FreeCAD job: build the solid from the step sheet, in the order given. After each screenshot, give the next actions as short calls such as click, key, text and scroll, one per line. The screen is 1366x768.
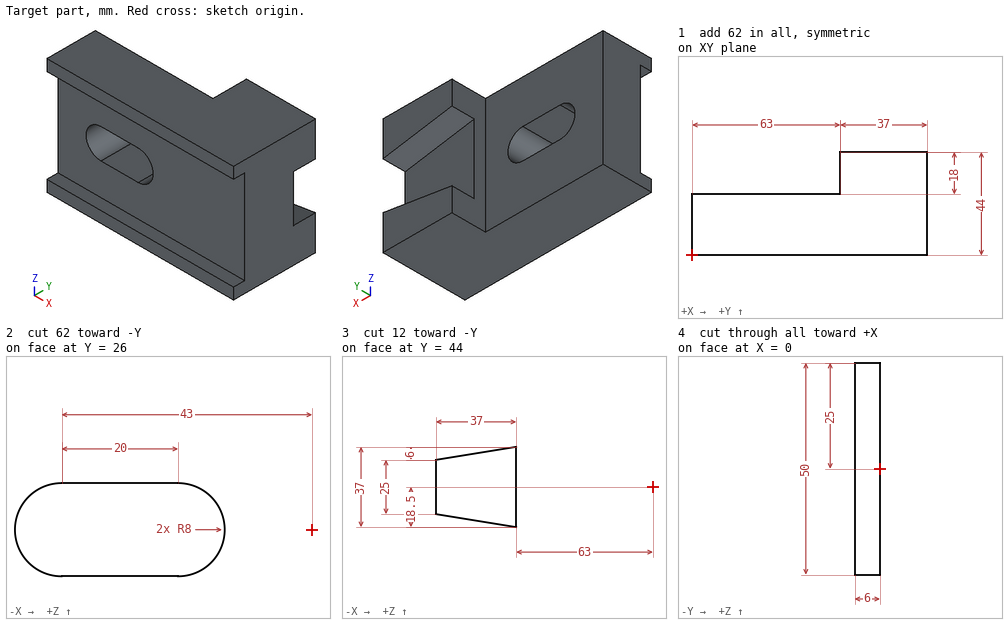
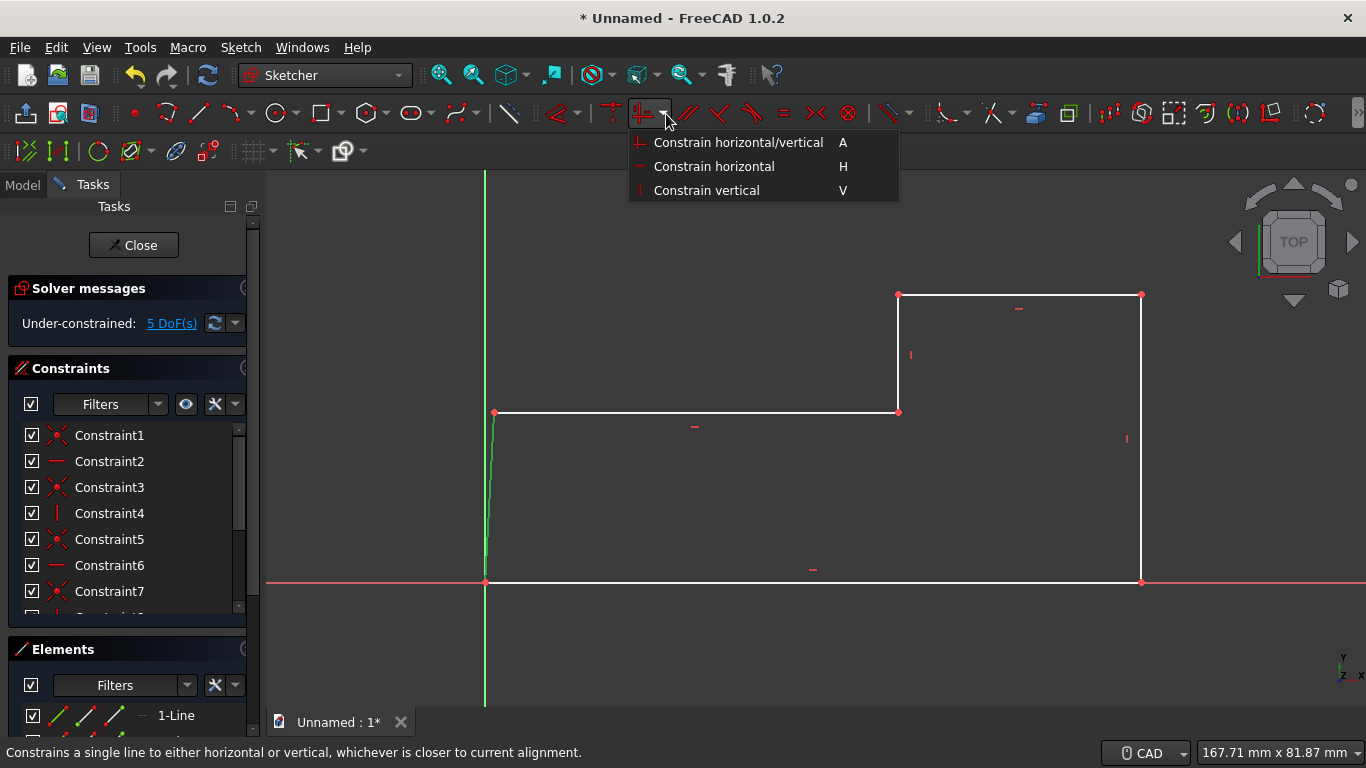
click(764, 190)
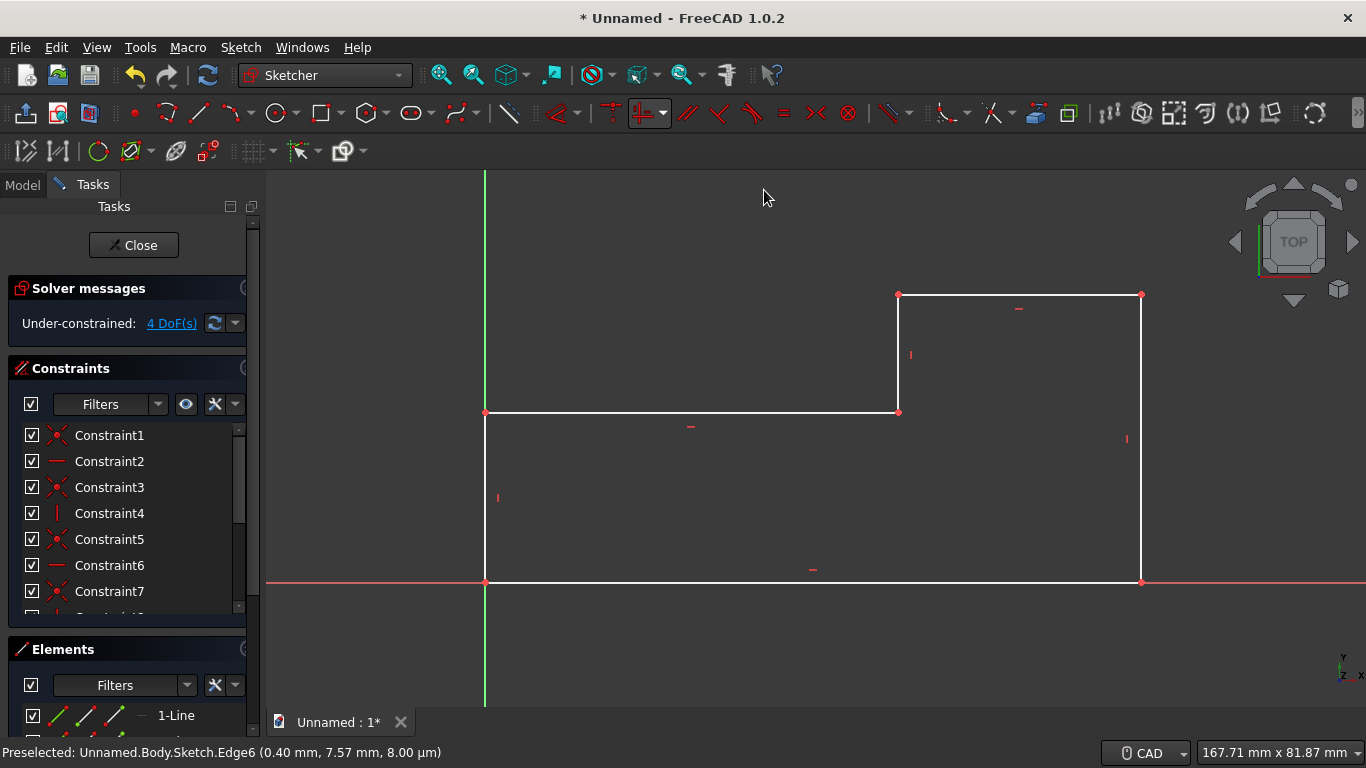
click(556, 114)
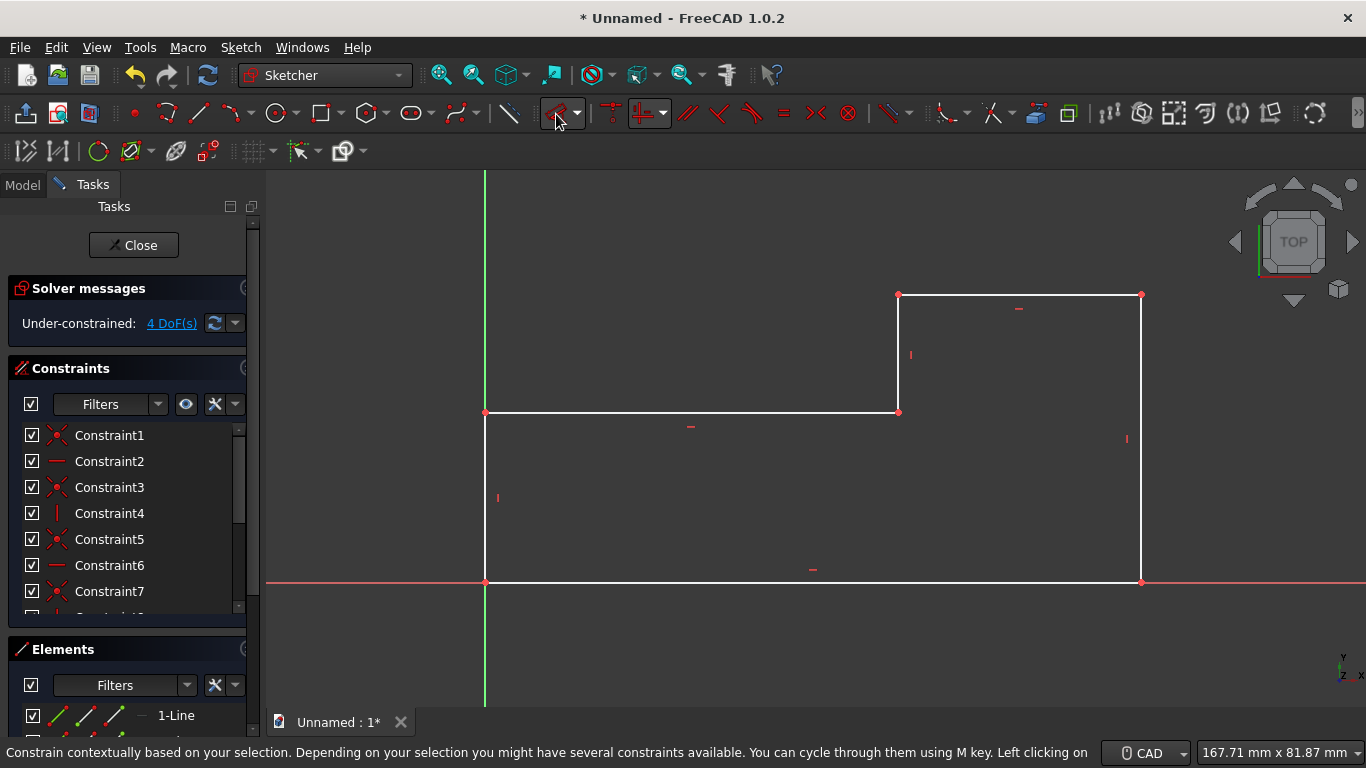
click(1141, 496)
click(1175, 439)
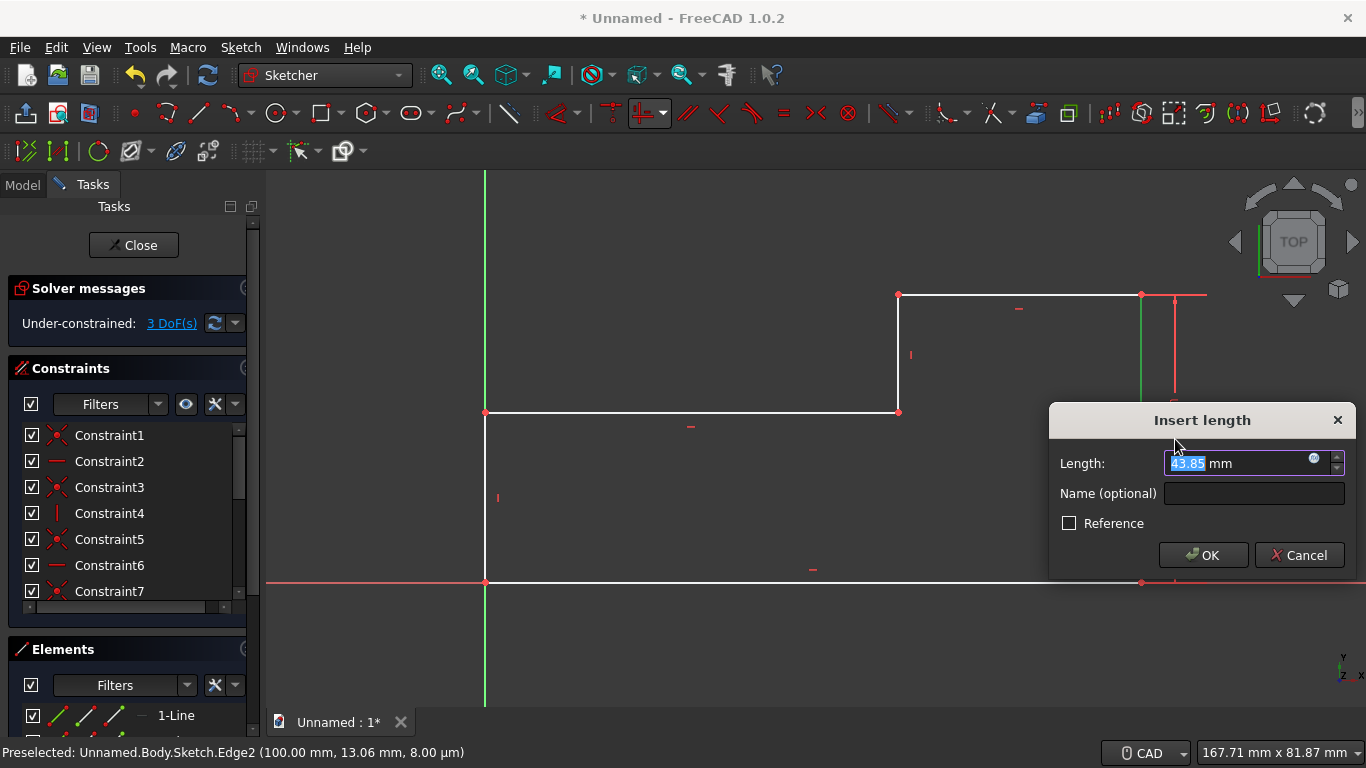
text(44)
key(Return)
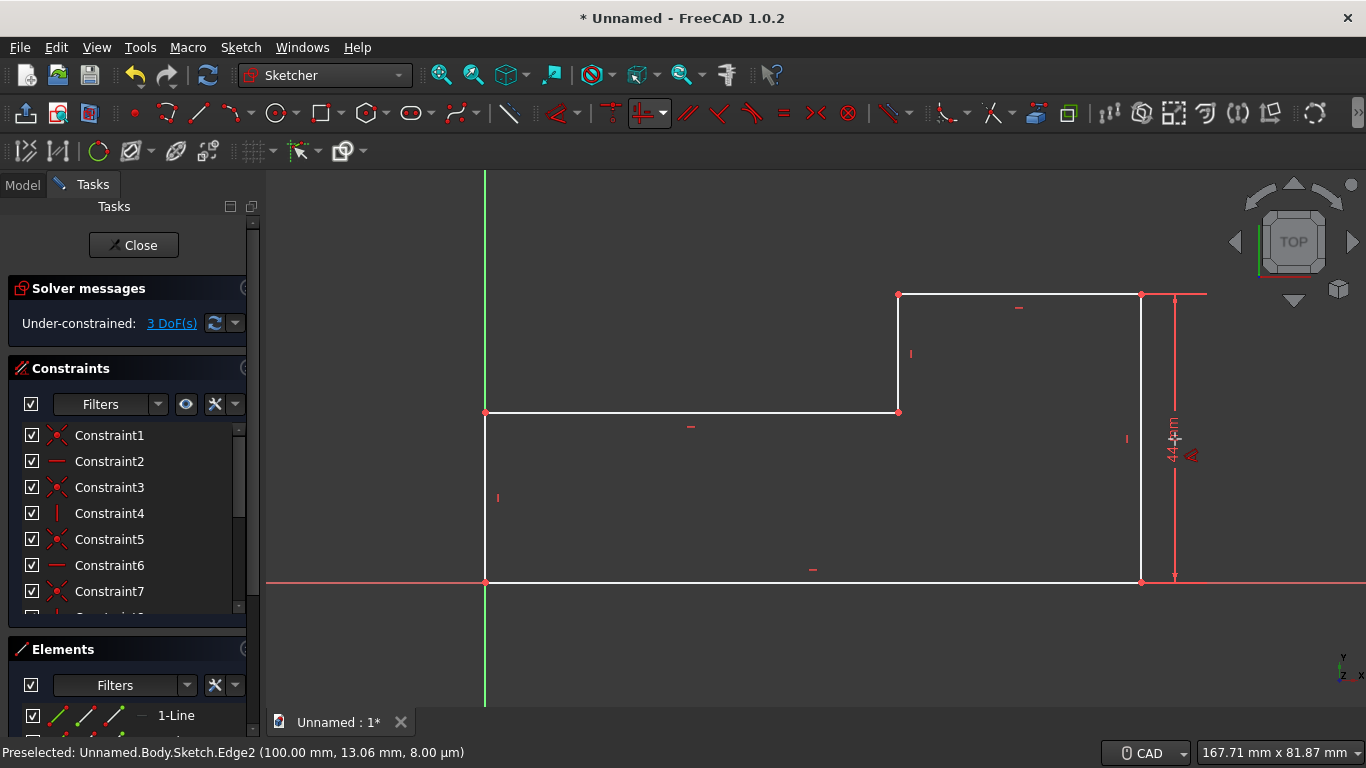
click(1068, 294)
click(1019, 260)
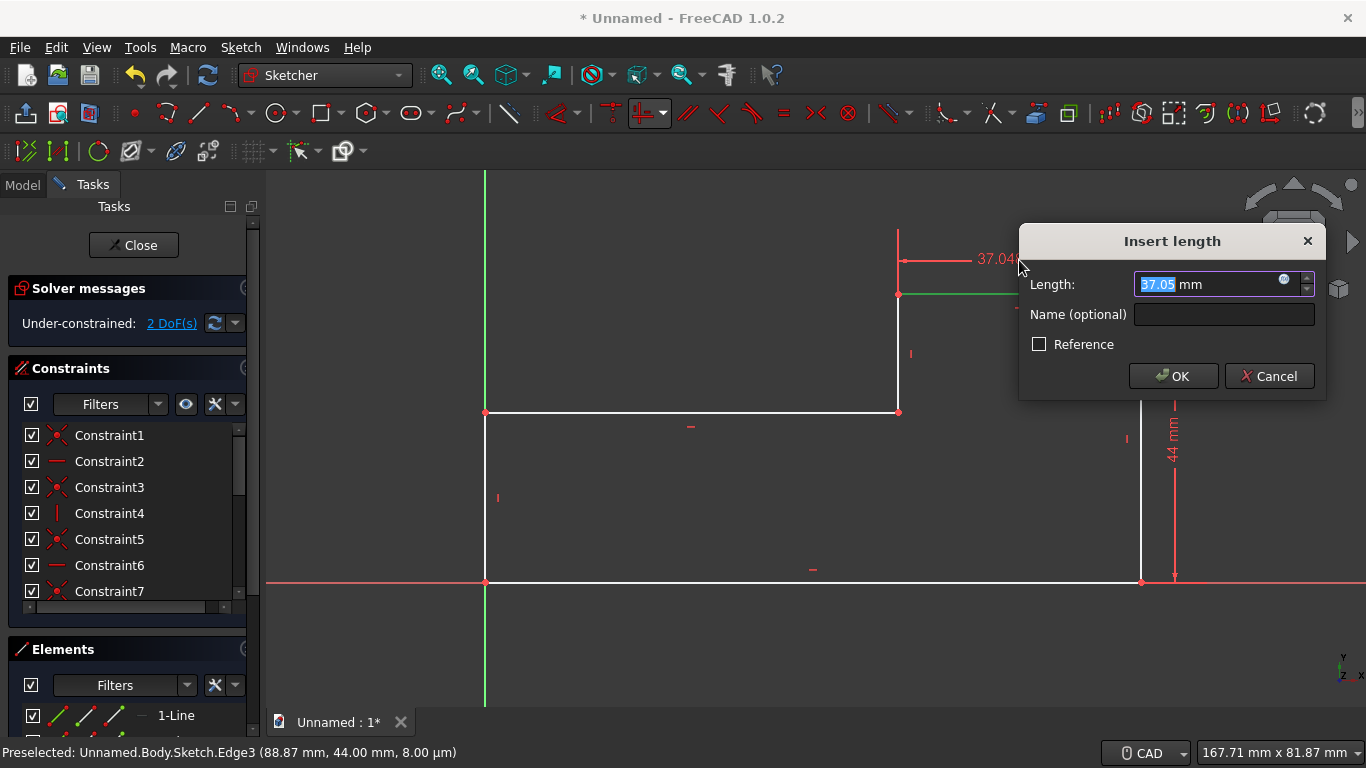
text(37)
key(Return)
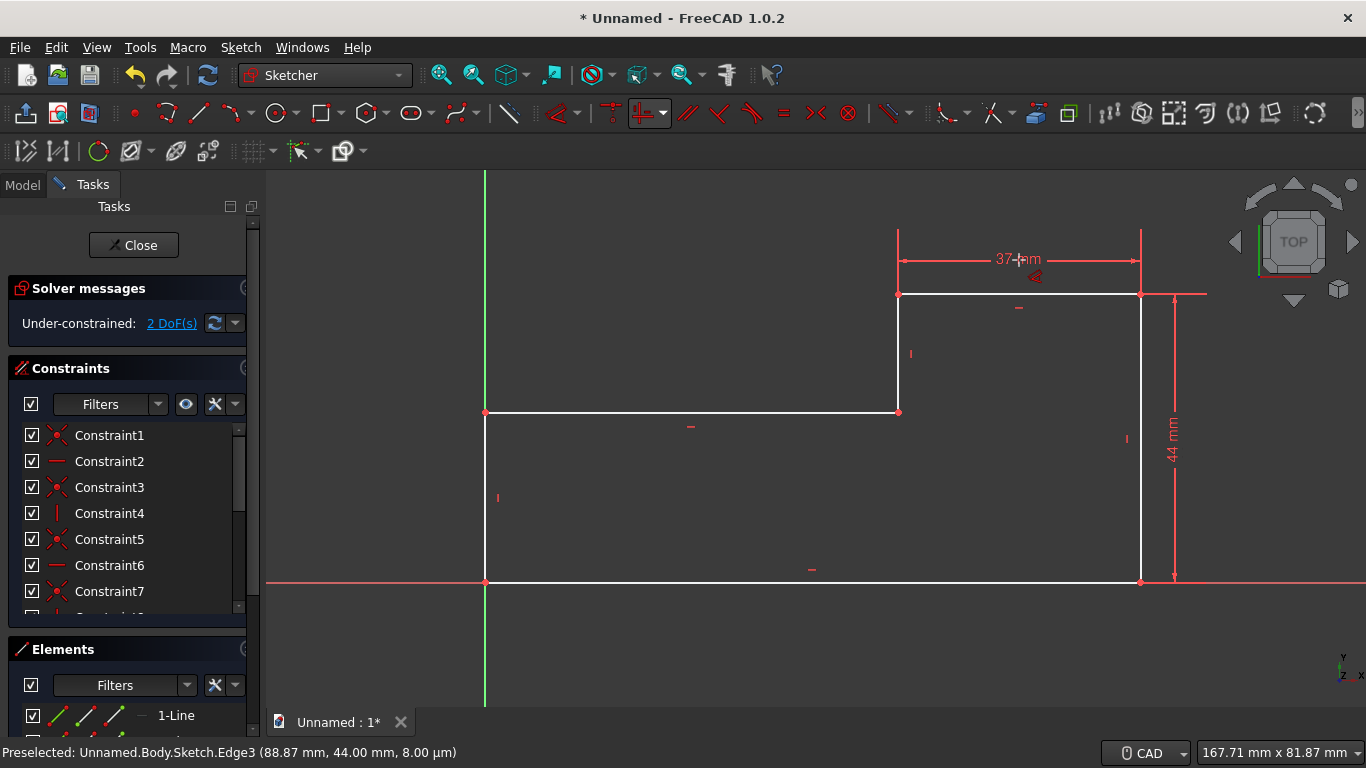
click(898, 330)
click(932, 354)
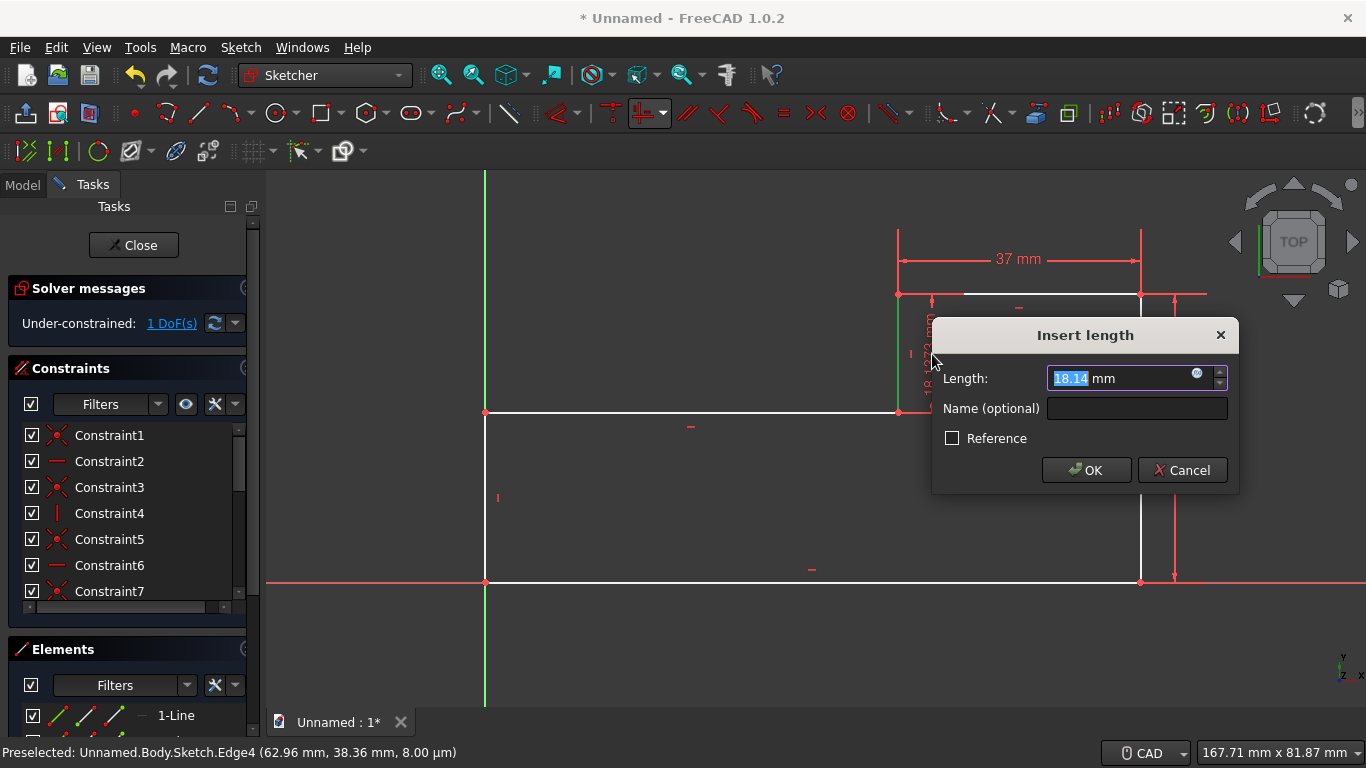
text(18)
key(Return)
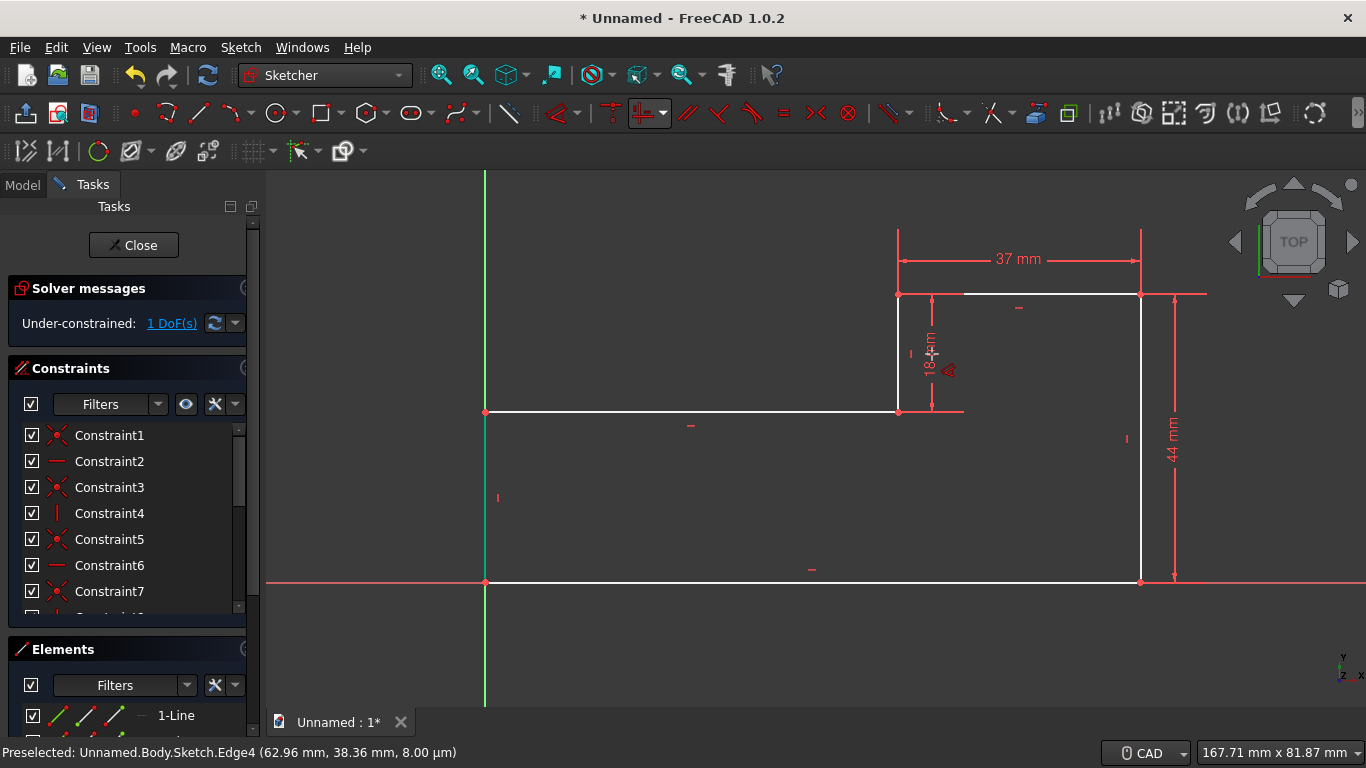
click(774, 412)
click(692, 378)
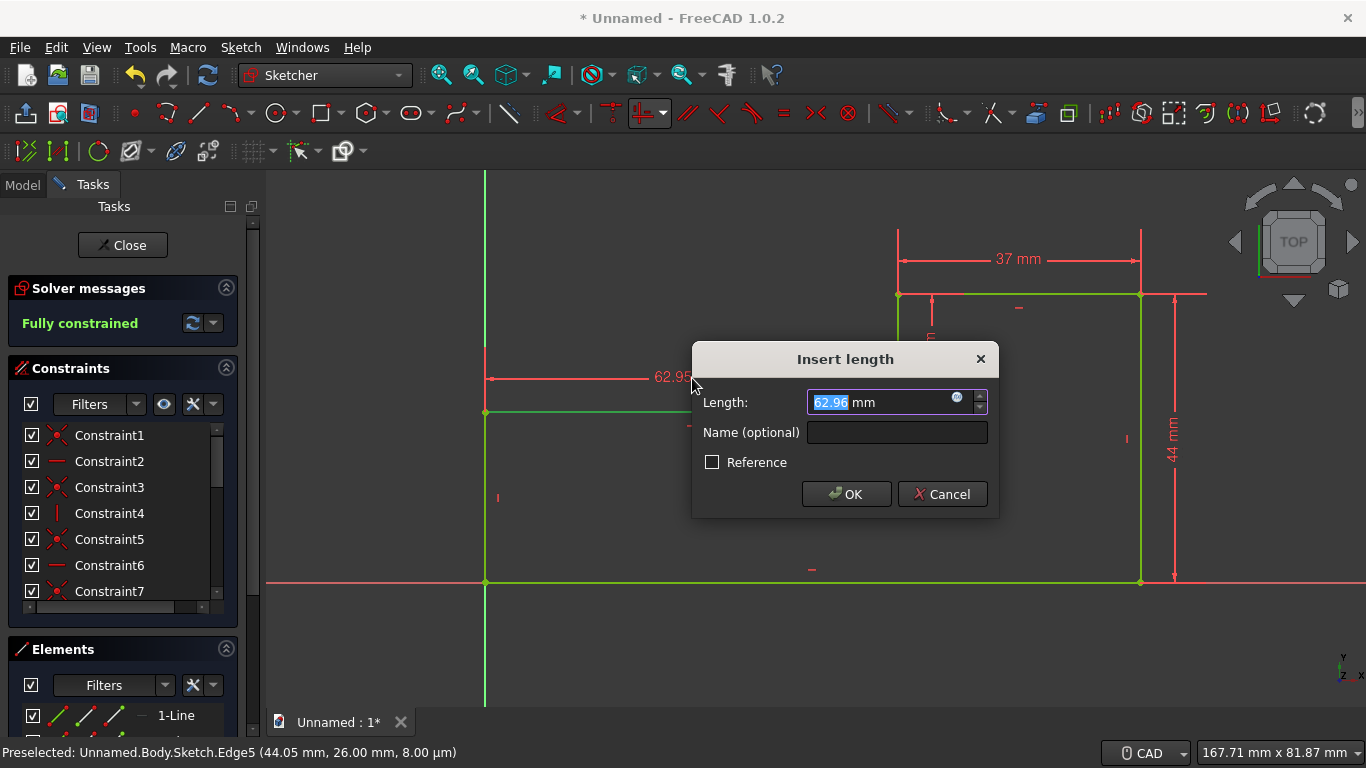
text(63)
key(Return)
key(Escape)